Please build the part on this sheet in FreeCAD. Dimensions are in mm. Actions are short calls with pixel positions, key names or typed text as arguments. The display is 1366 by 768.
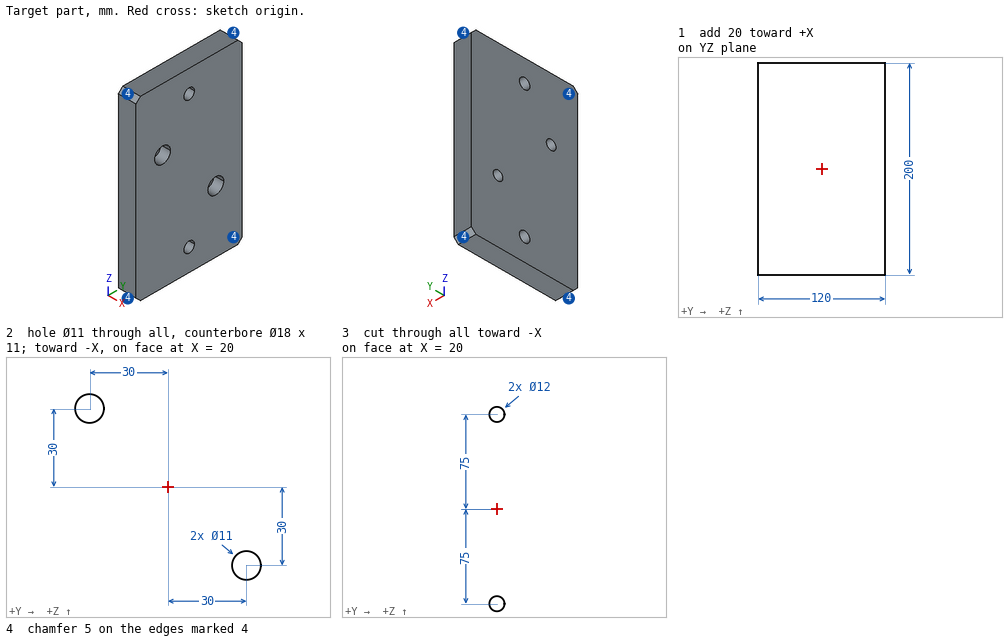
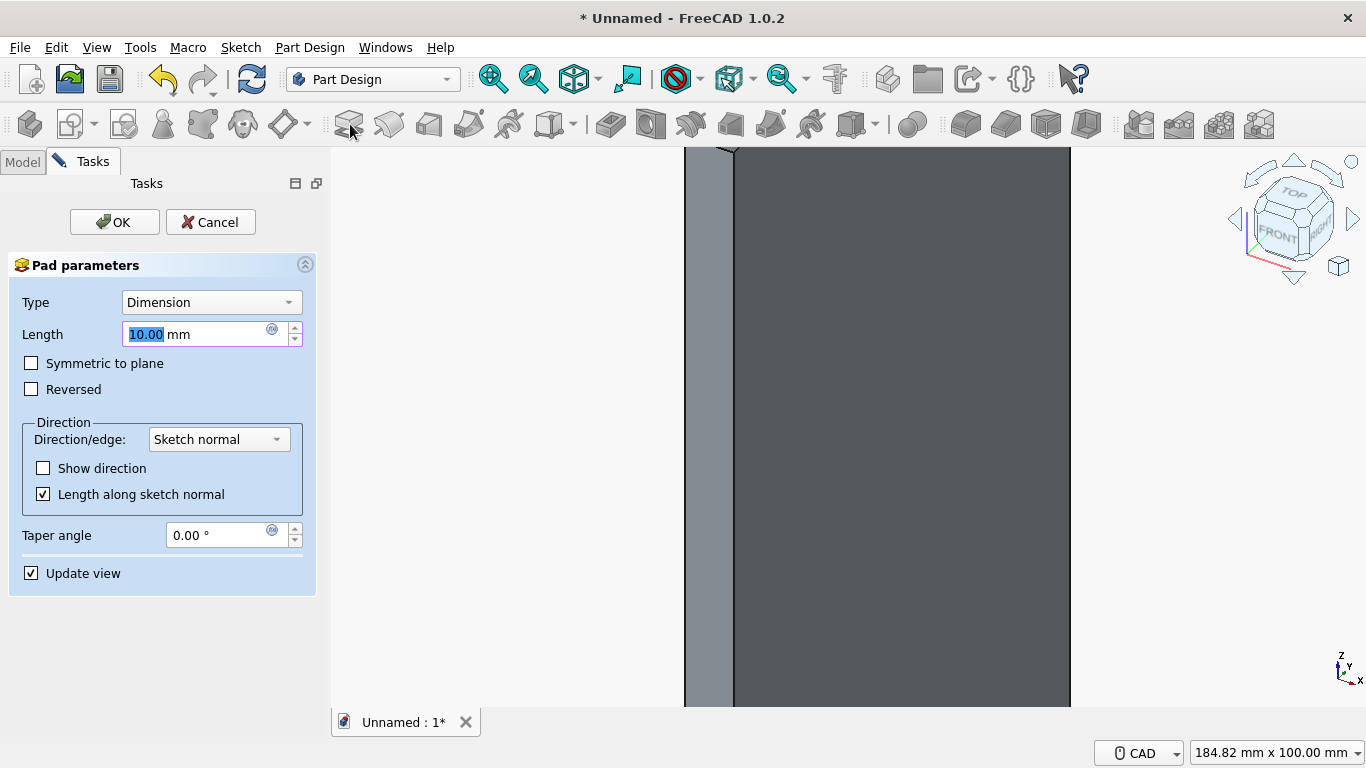
text(20)
key(Tab)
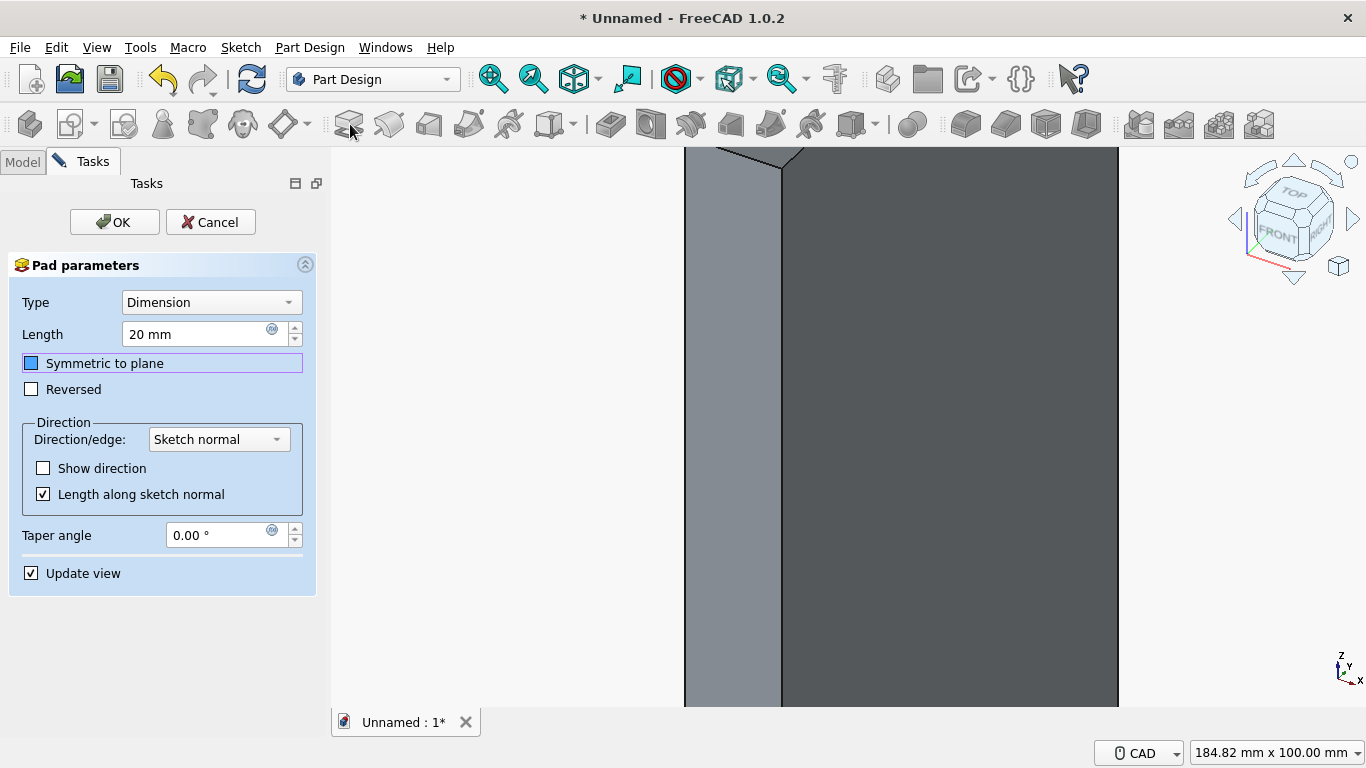
click(115, 222)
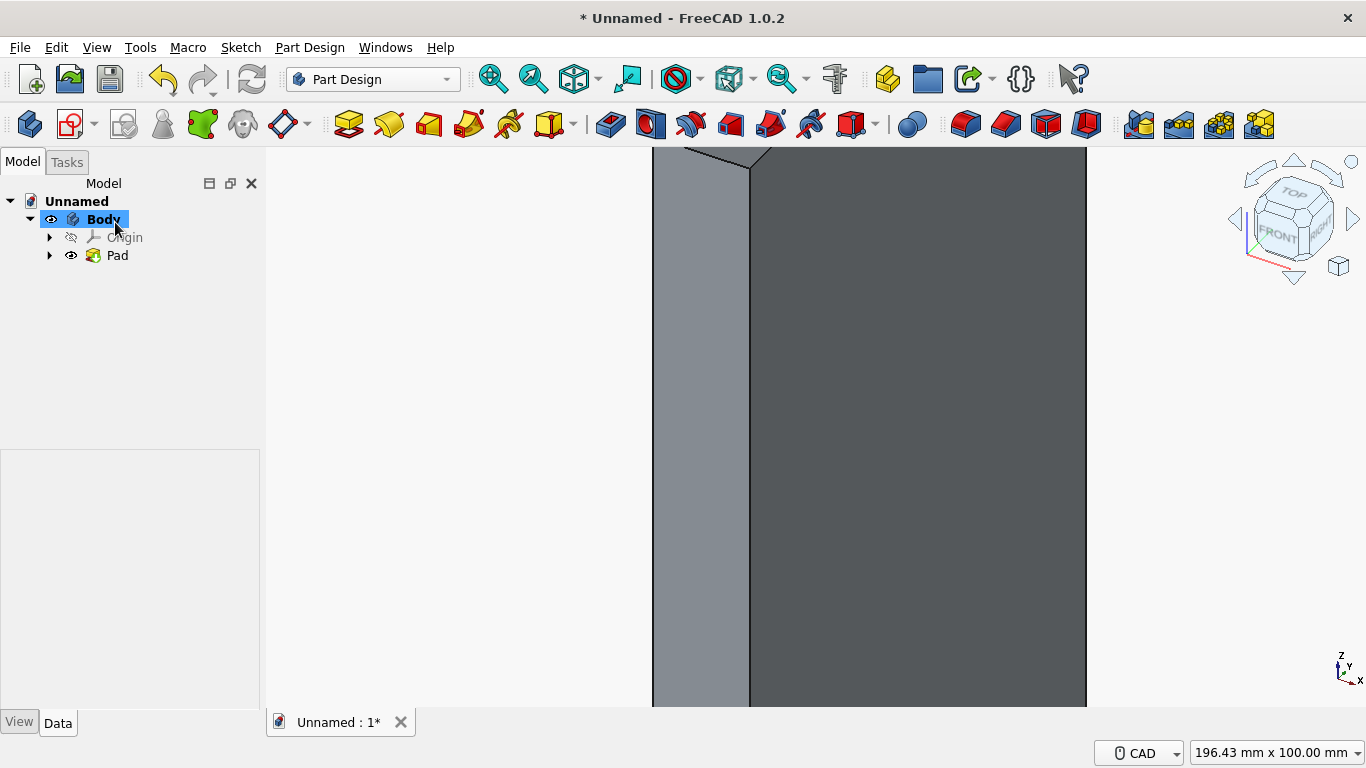
click(494, 80)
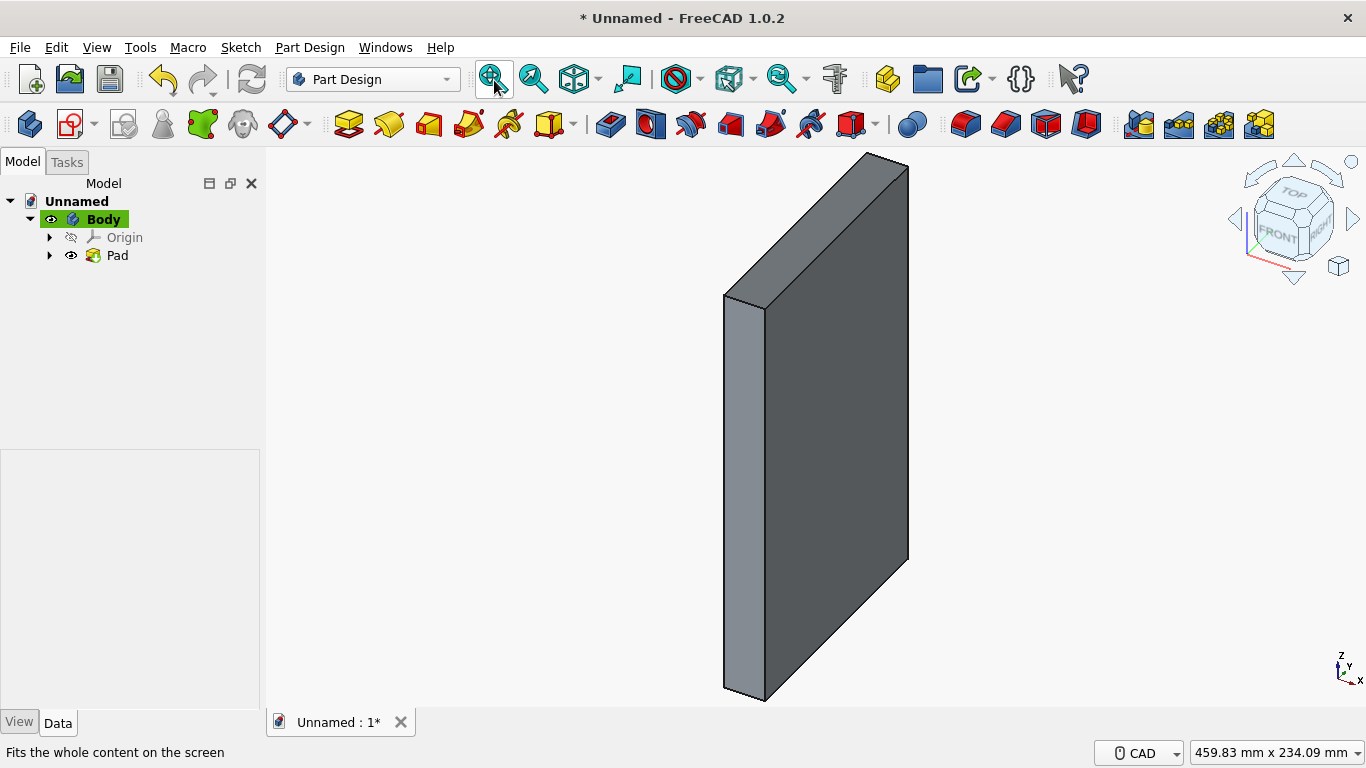
click(837, 433)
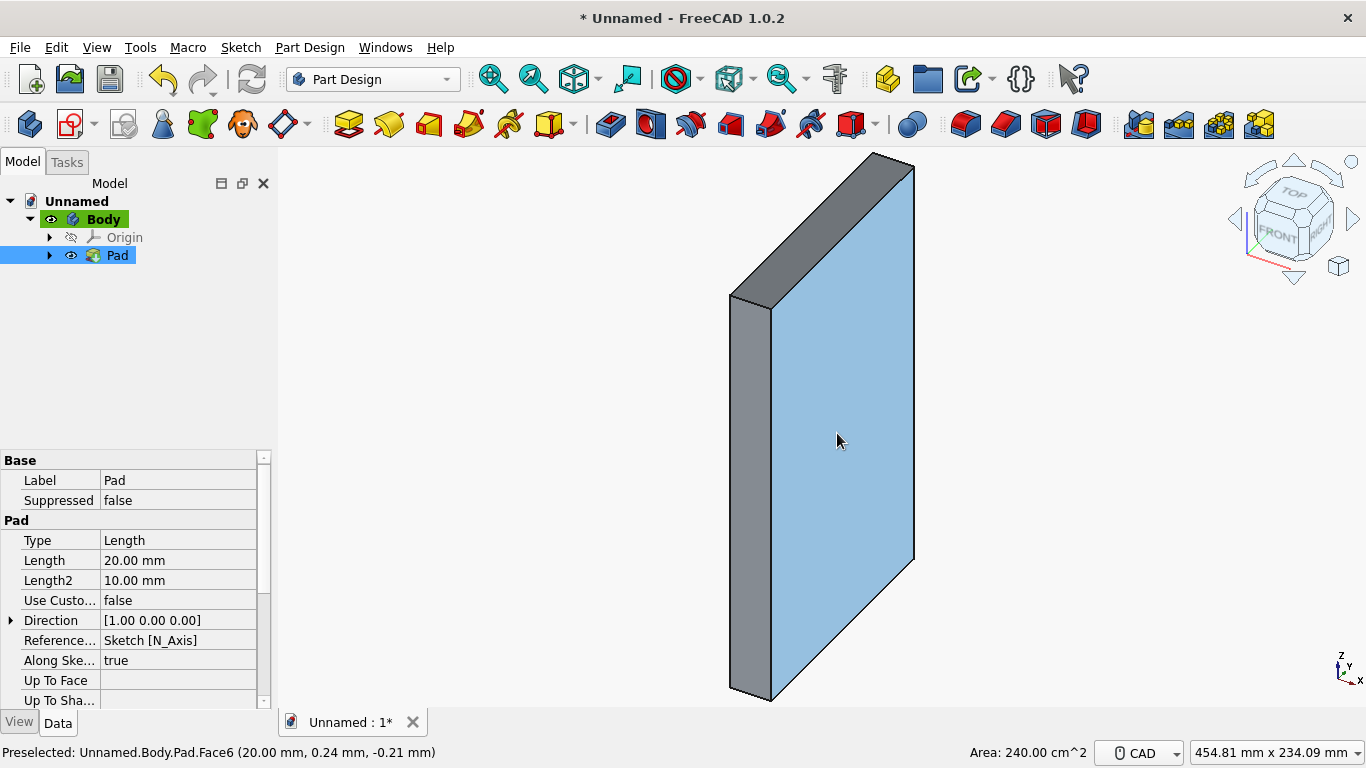
click(70, 124)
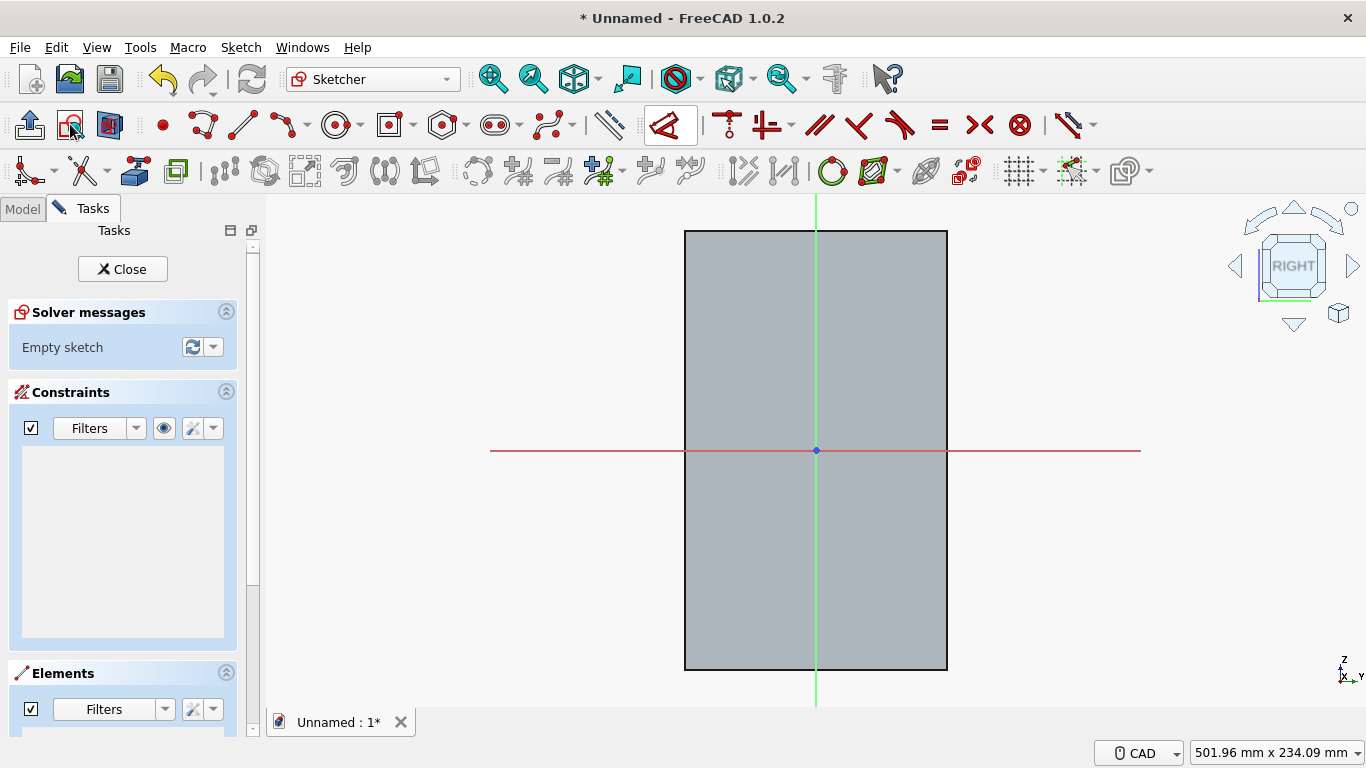
scroll(872, 450, up, 4)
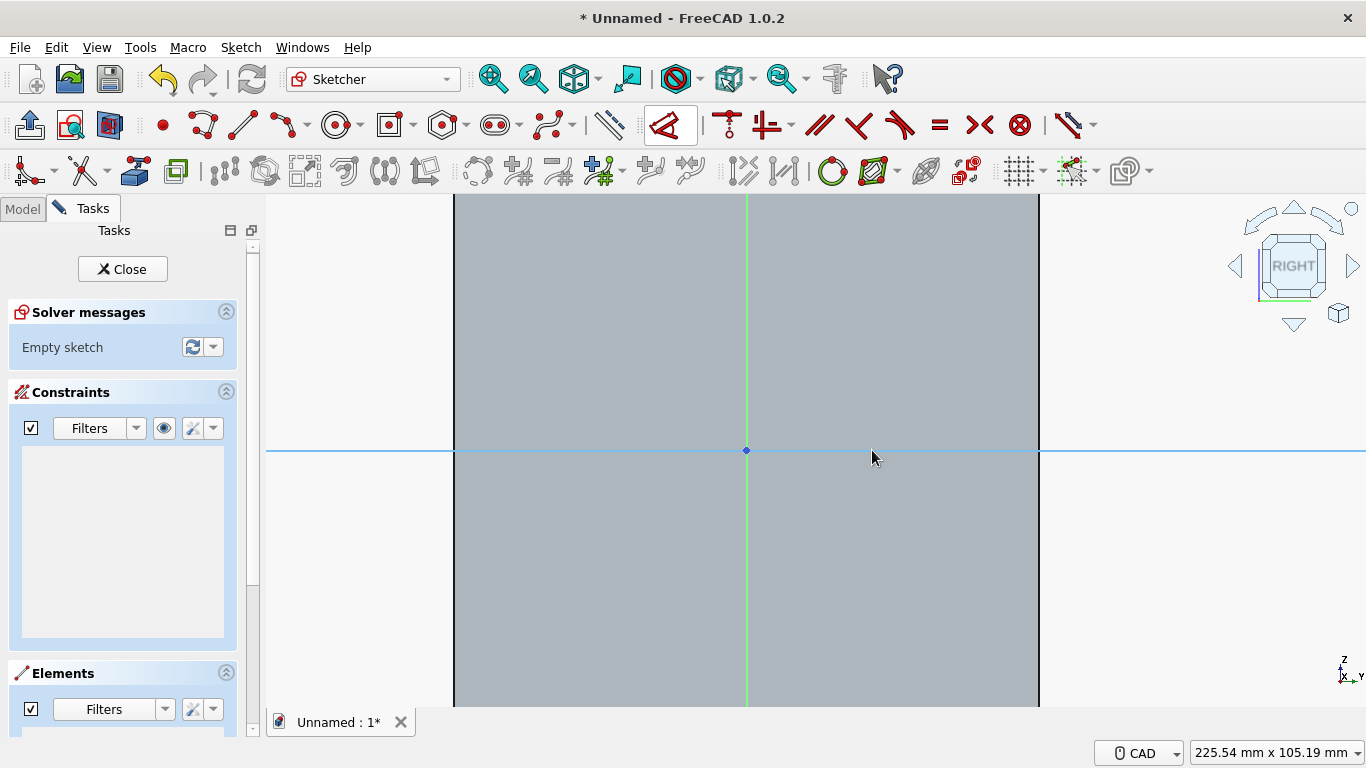
key(g)
key(c)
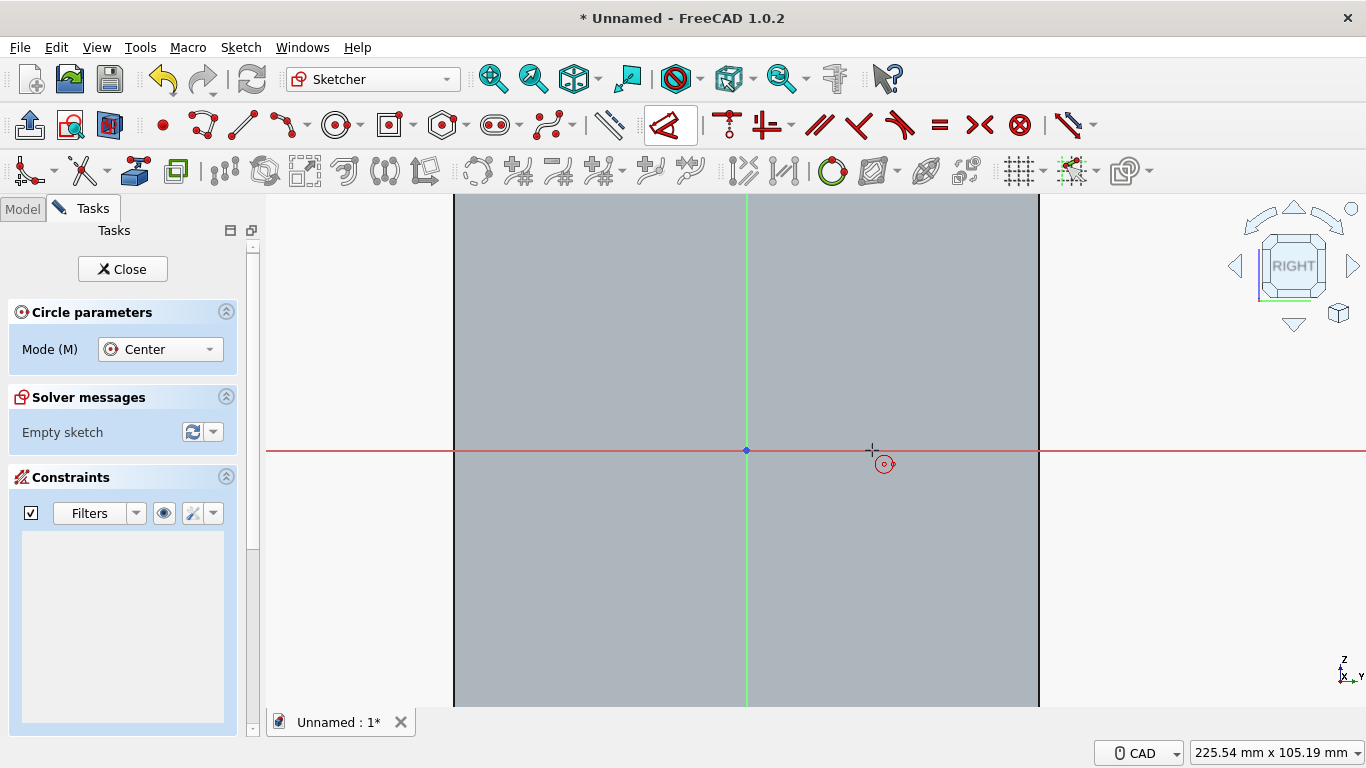
click(893, 597)
move(912, 578)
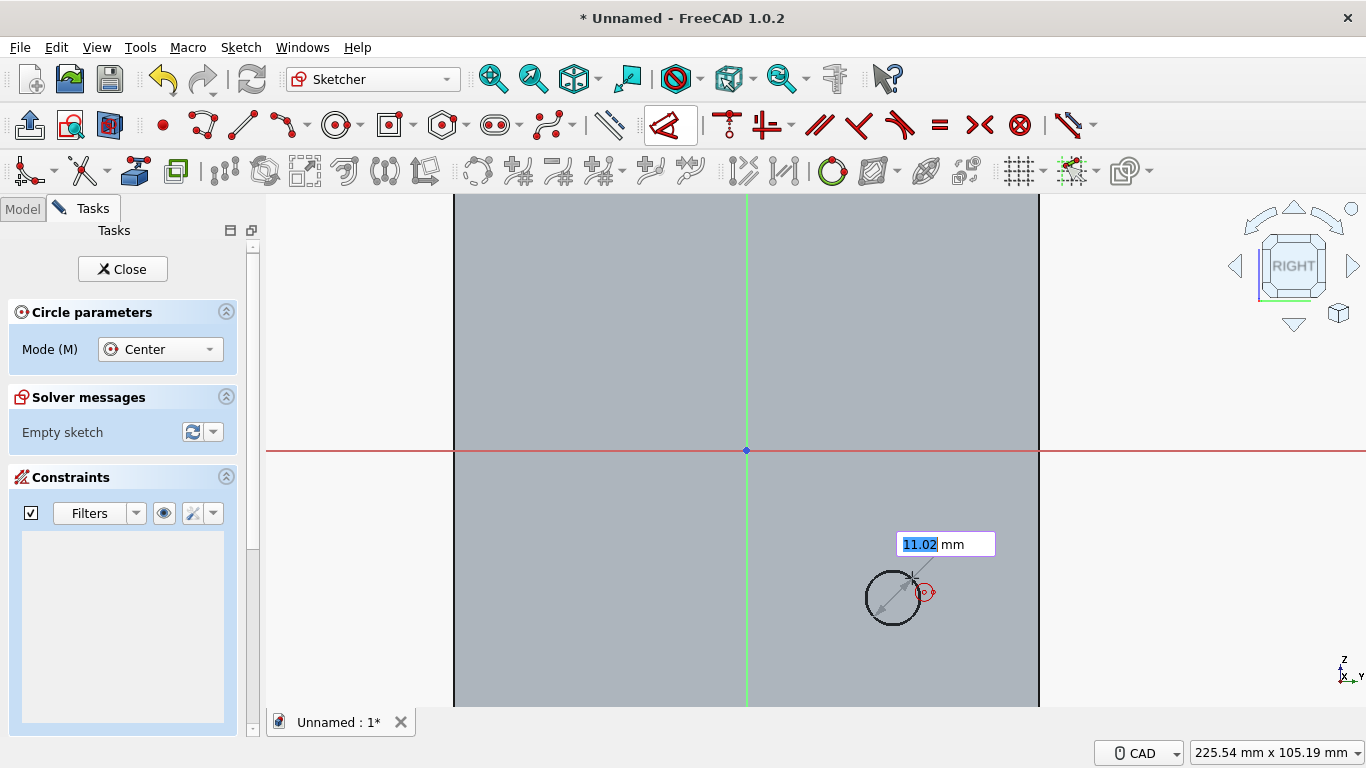
text(11)
key(Return)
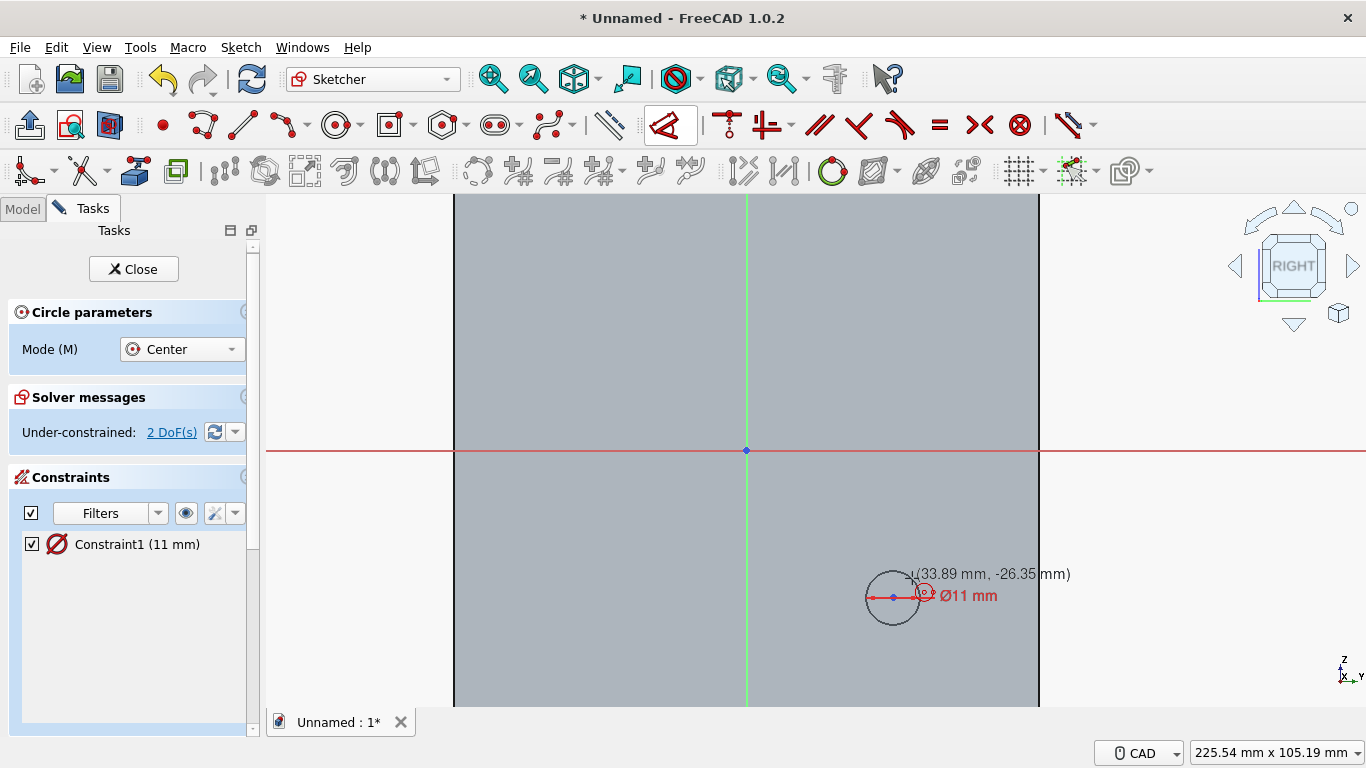
click(600, 304)
move(619, 285)